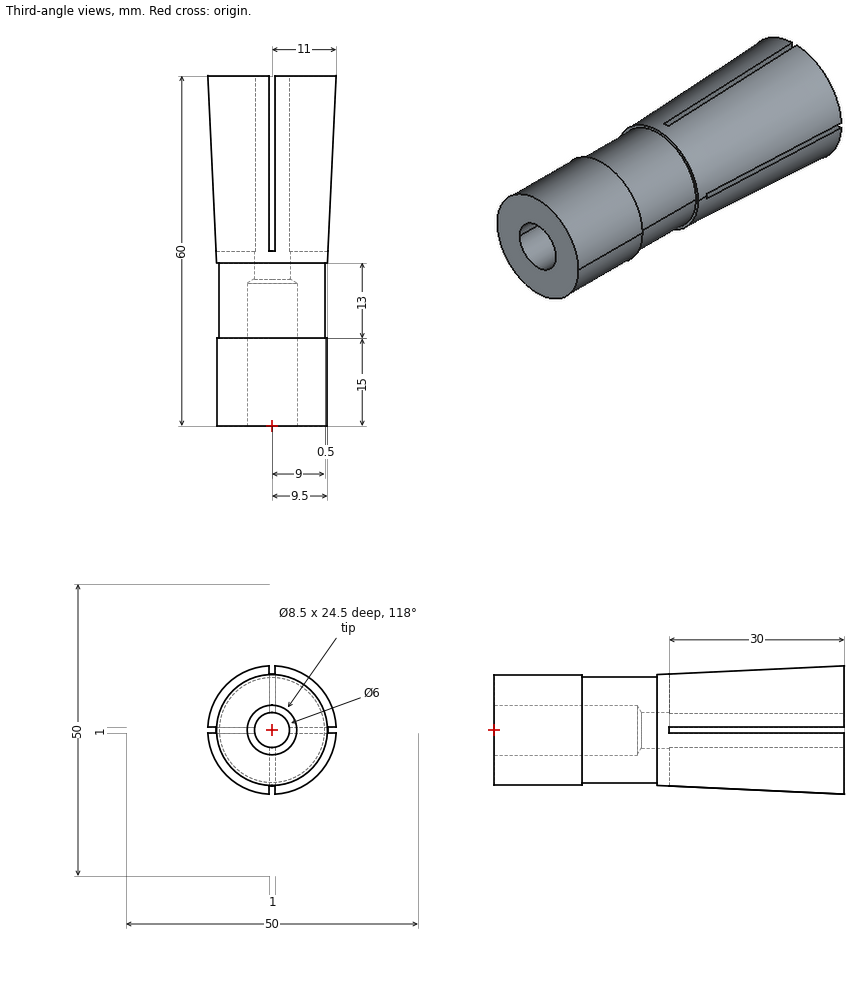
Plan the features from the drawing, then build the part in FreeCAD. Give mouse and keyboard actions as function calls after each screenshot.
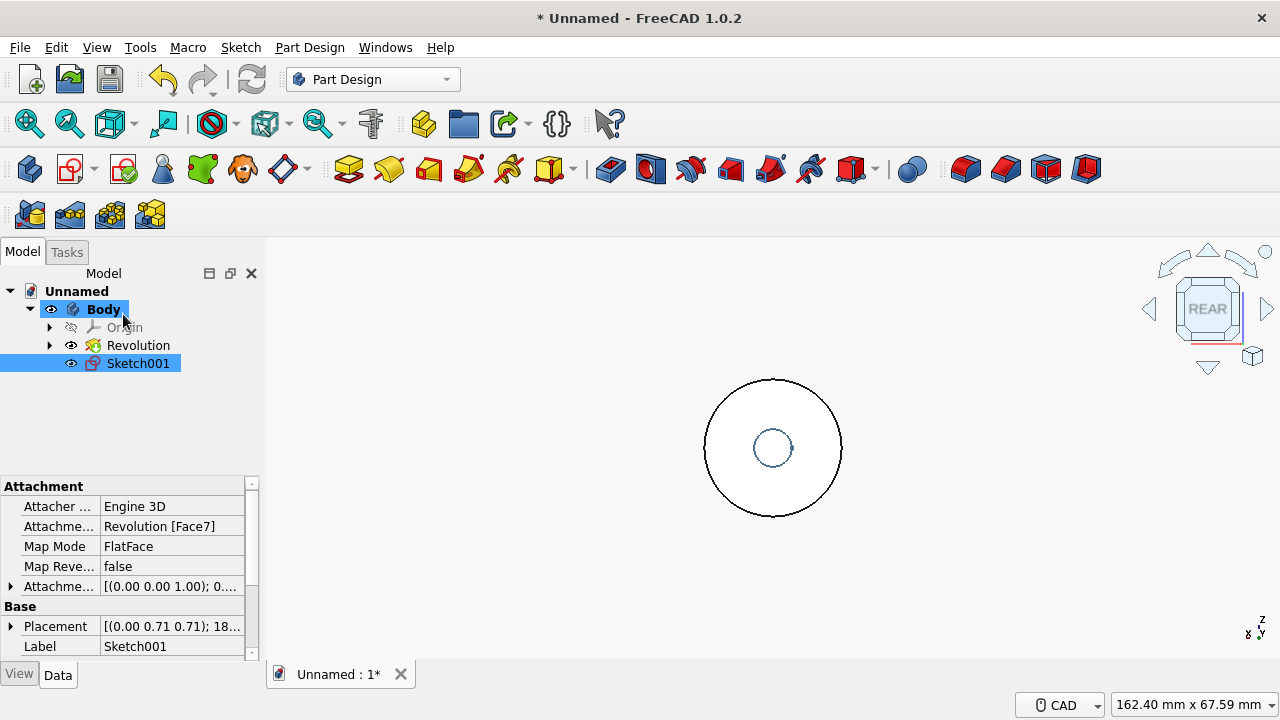
click(612, 170)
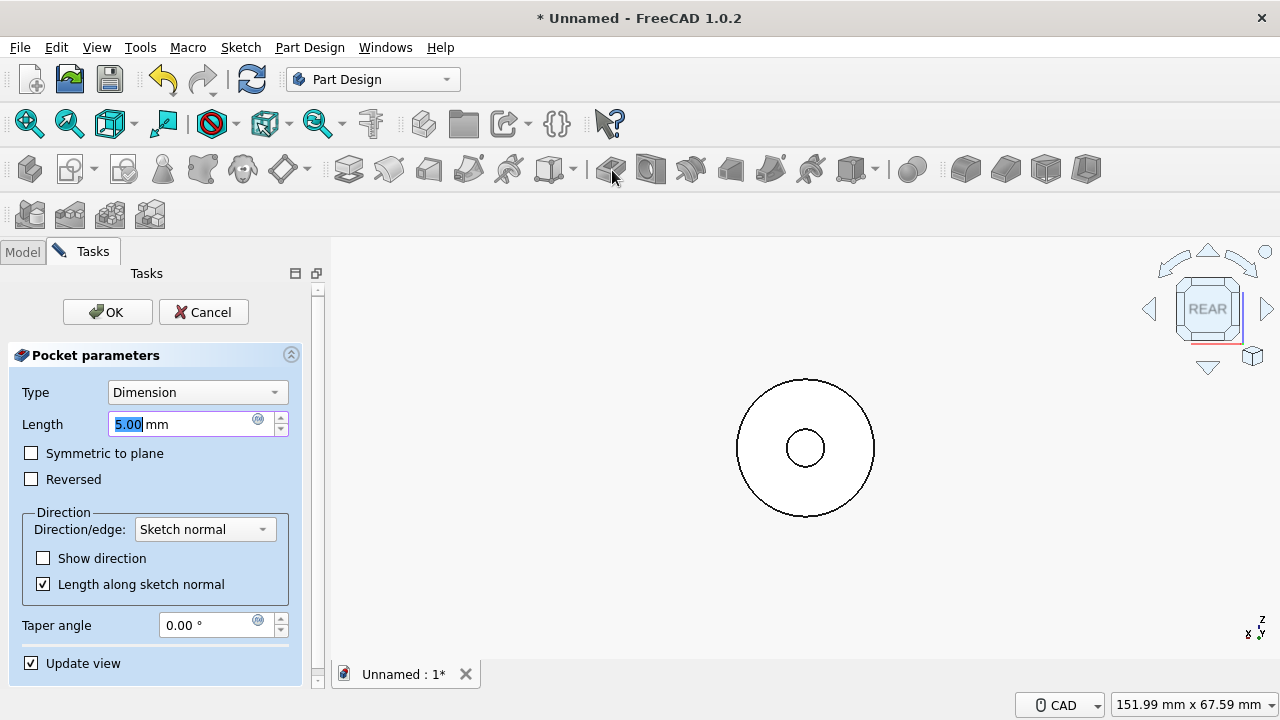
click(198, 392)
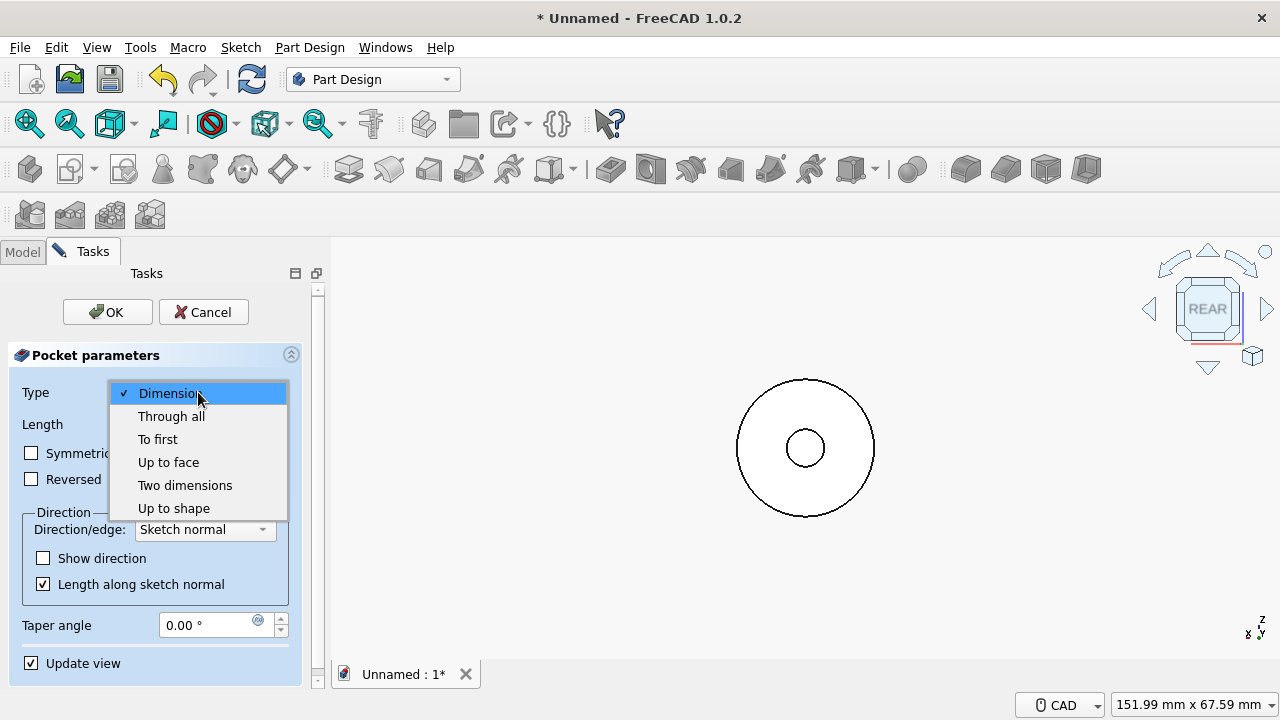
click(198, 416)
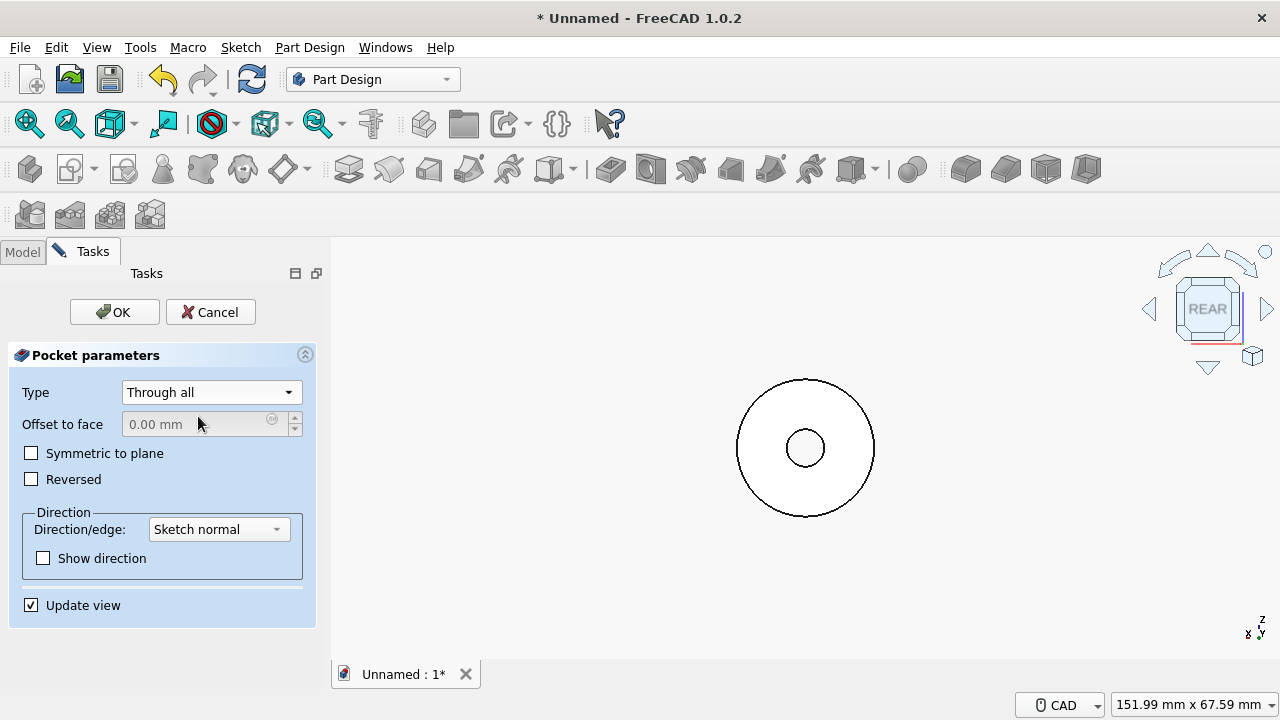
click(115, 312)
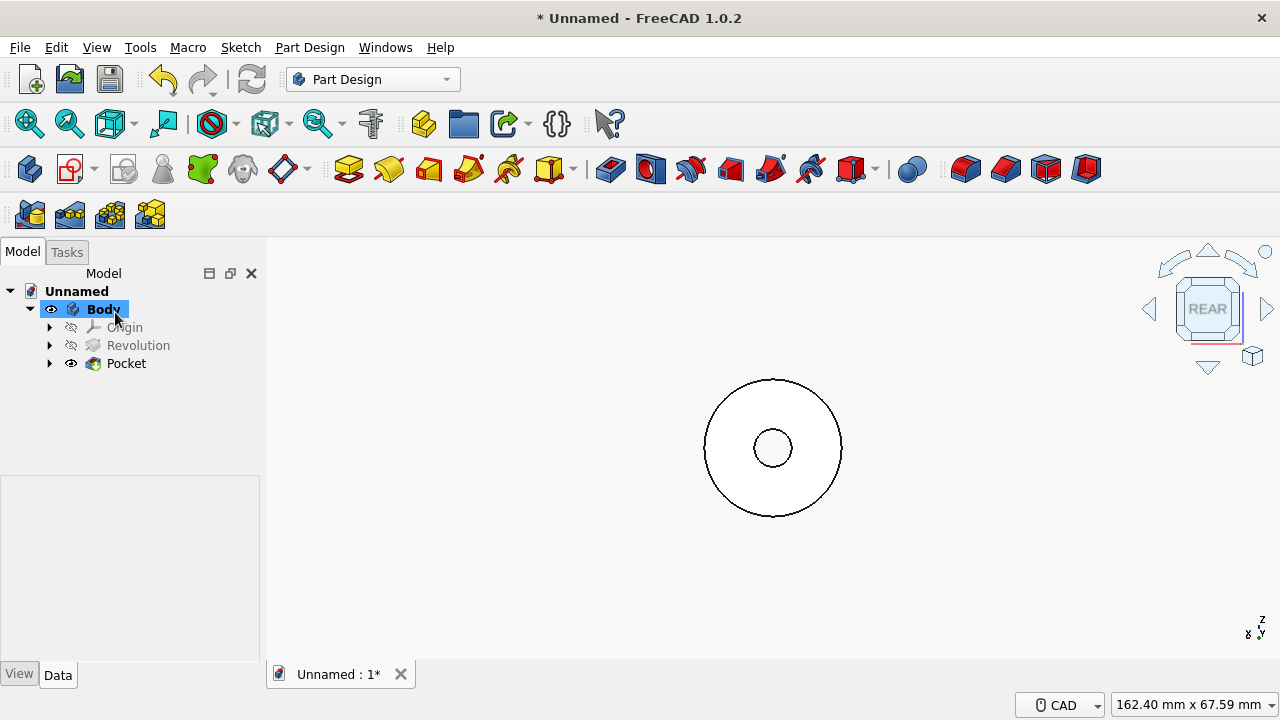
click(30, 124)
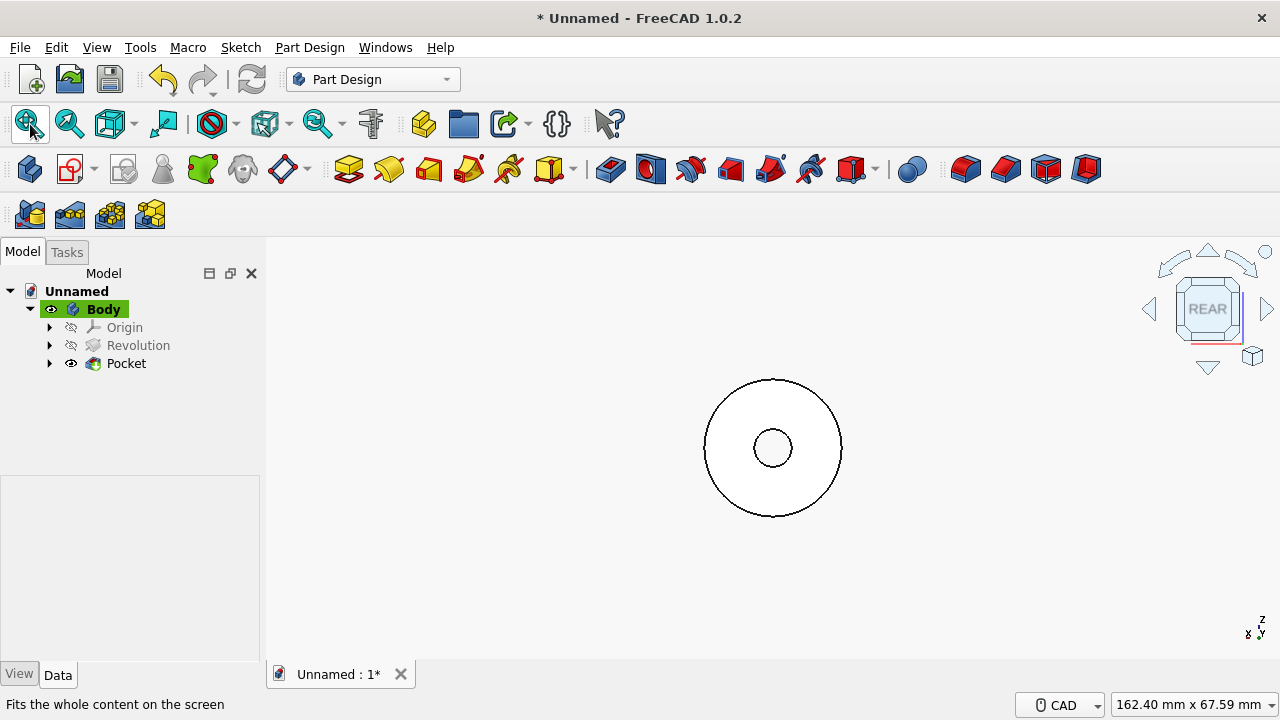
click(70, 170)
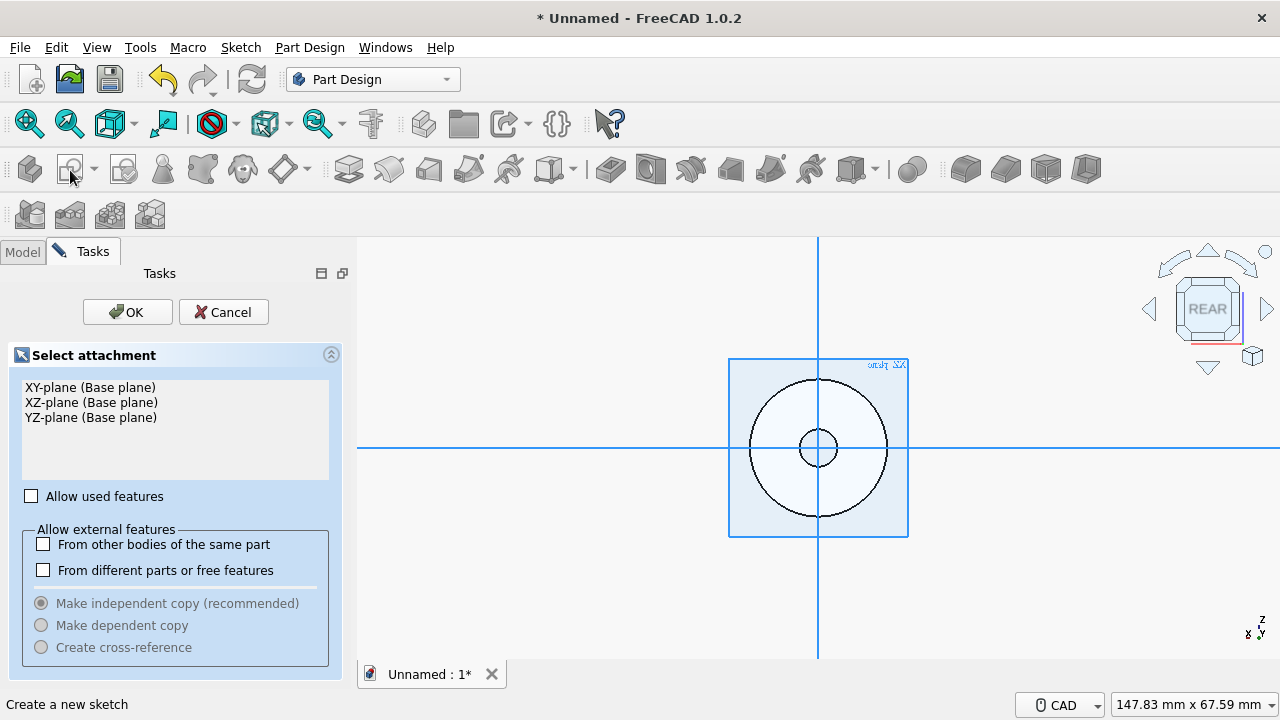
click(82, 402)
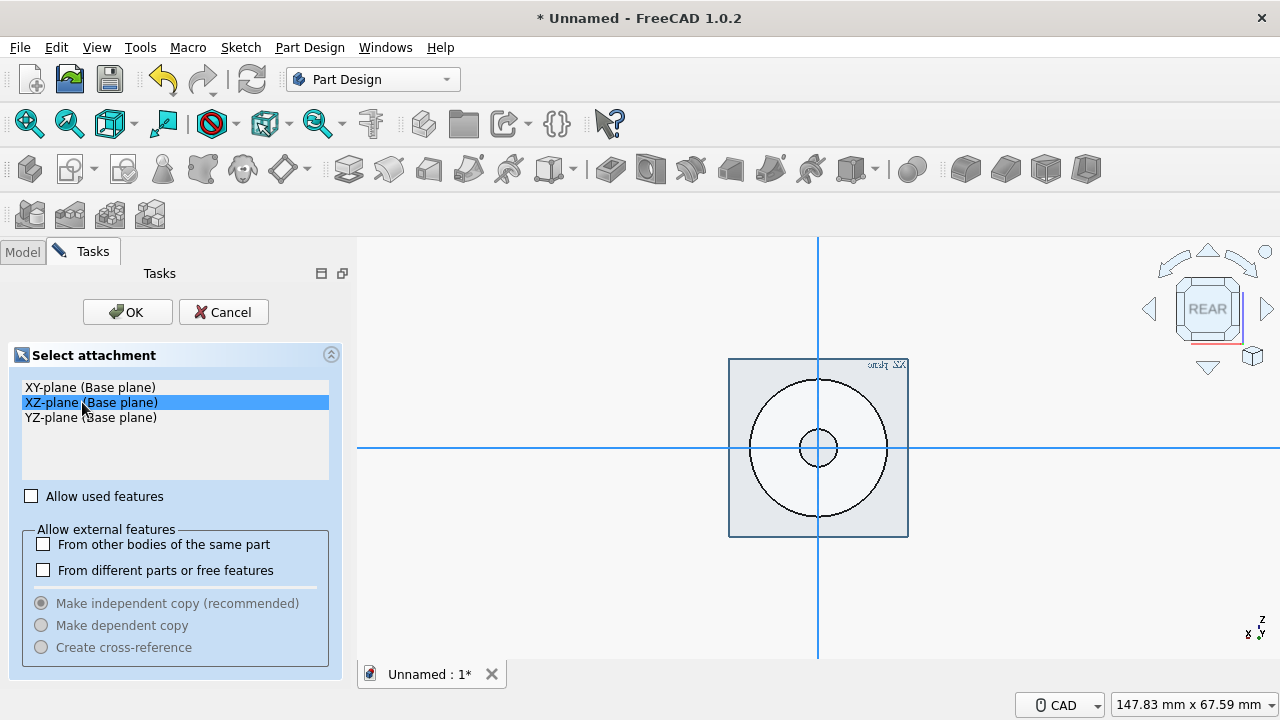
click(128, 312)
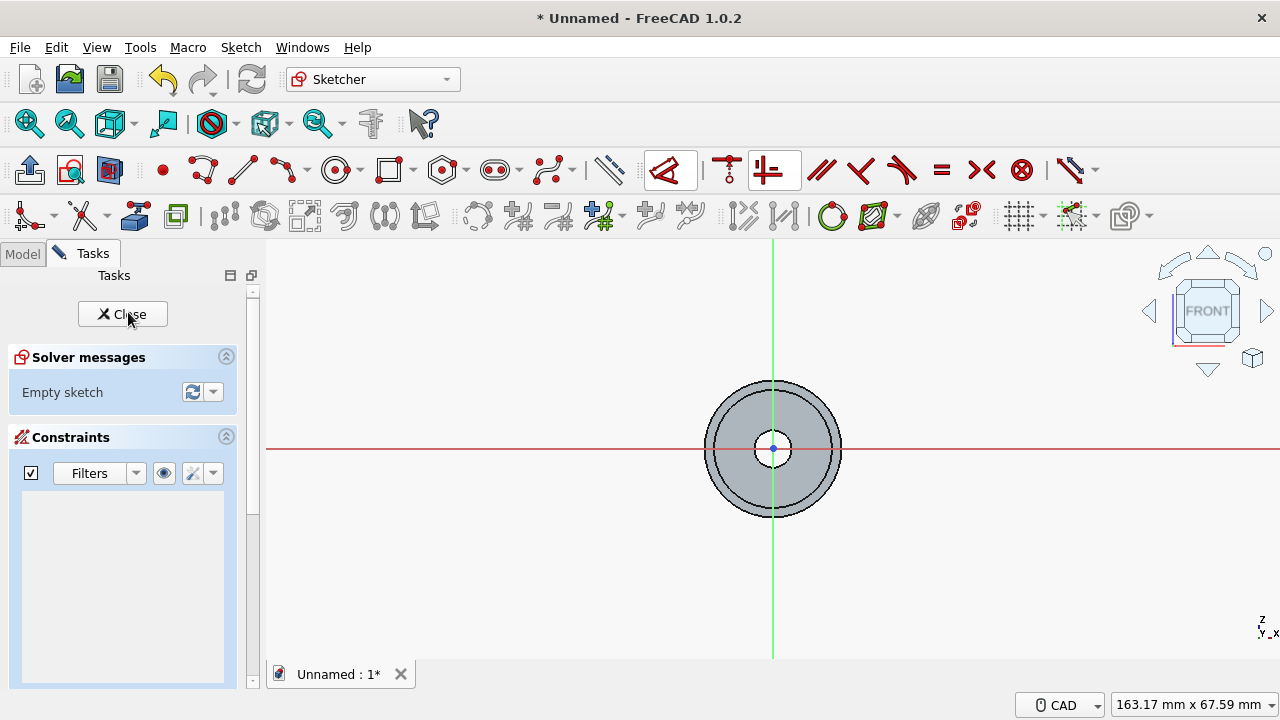
scroll(790, 449, up, 8)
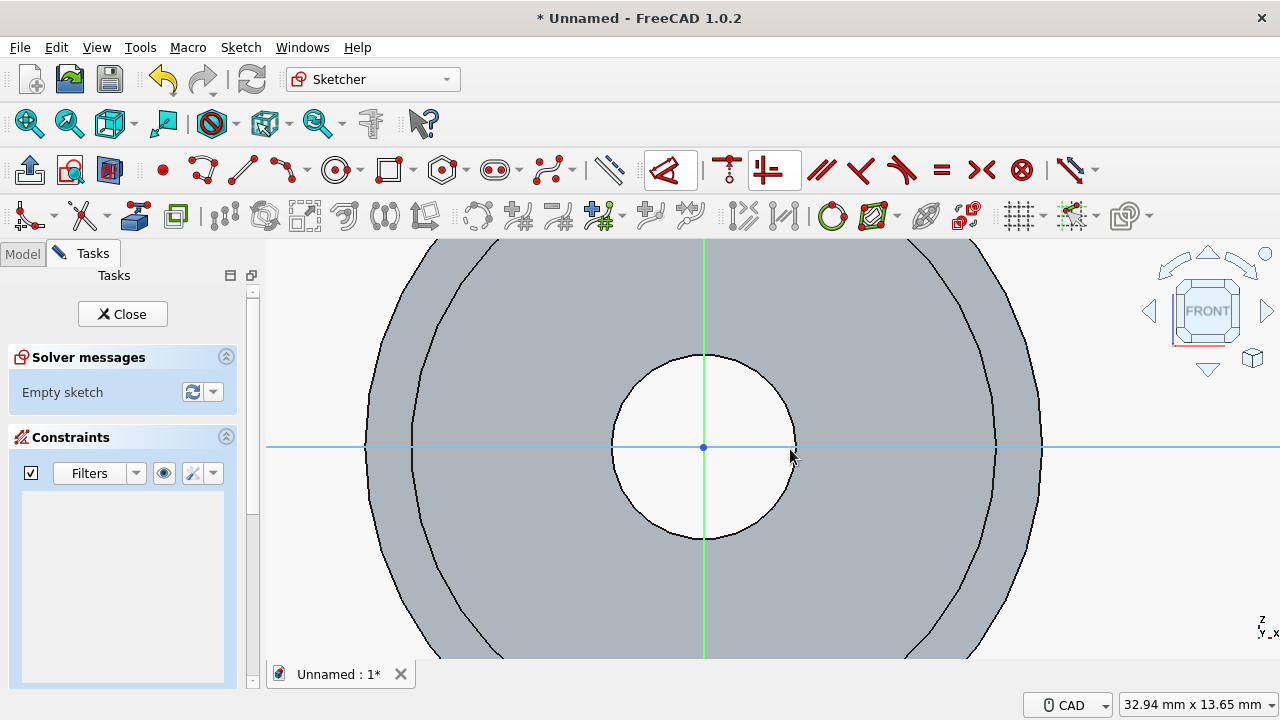
click(336, 170)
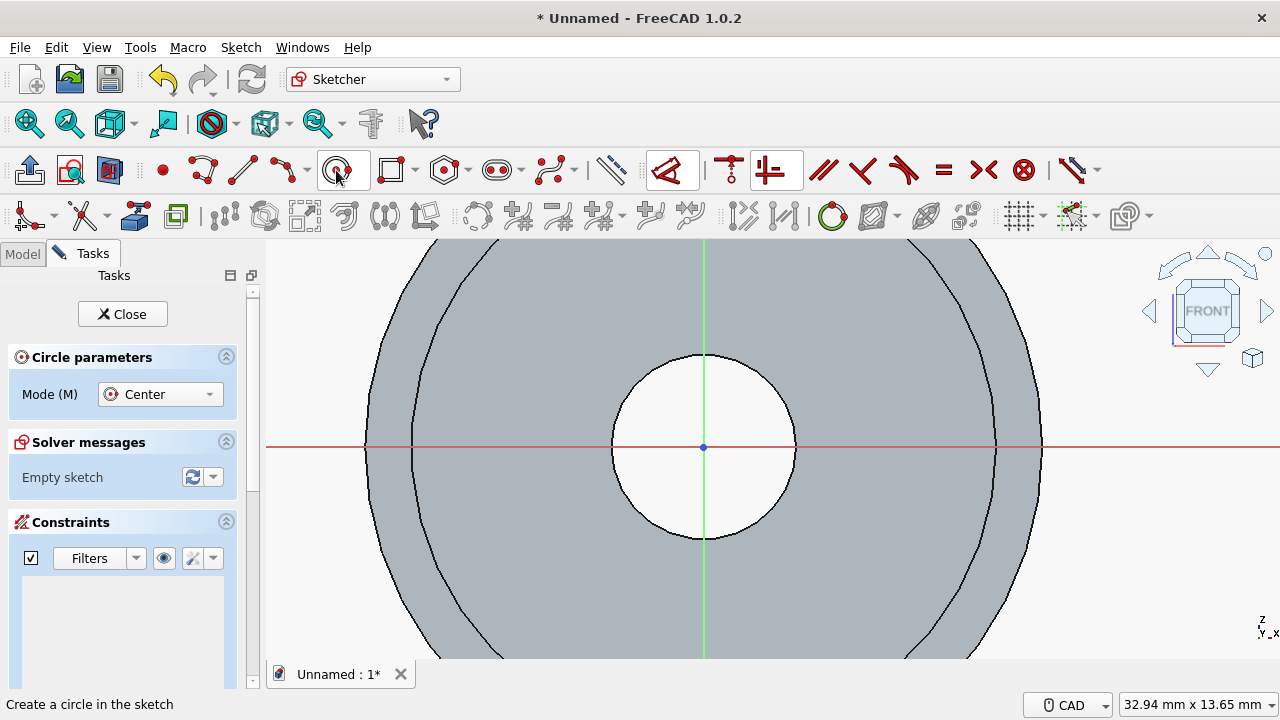
click(704, 447)
move(796, 355)